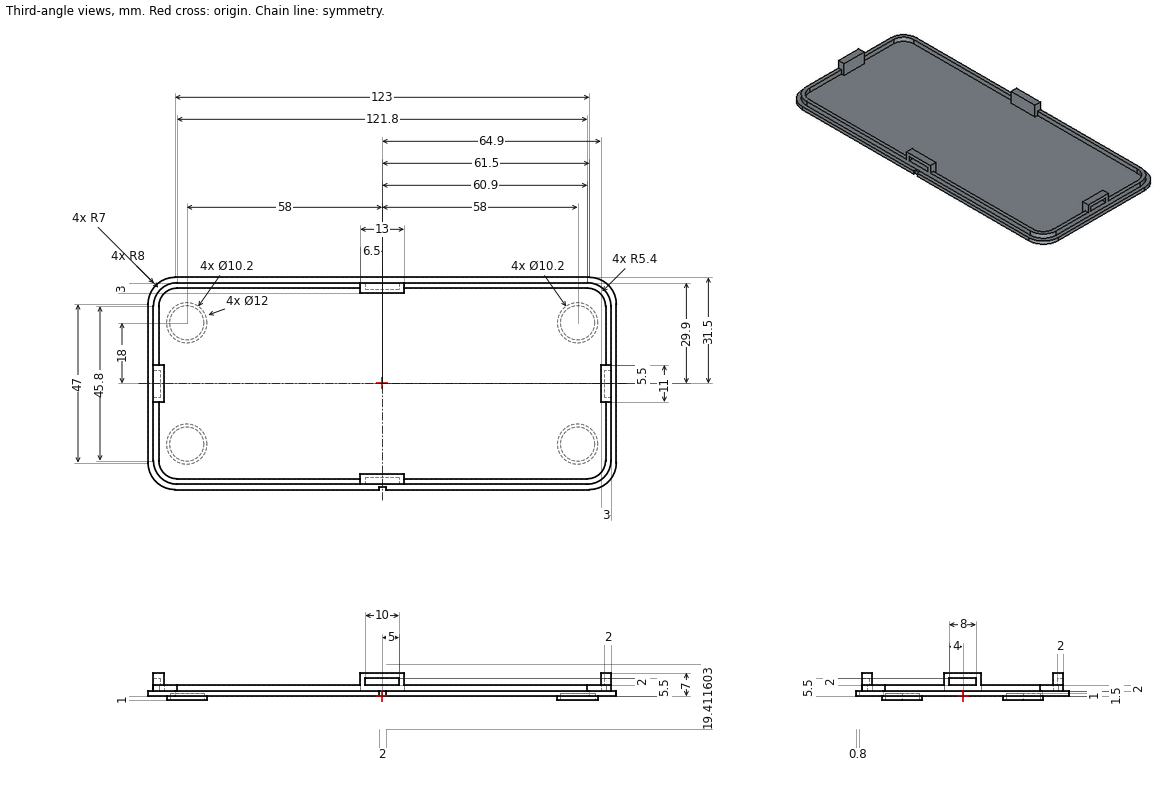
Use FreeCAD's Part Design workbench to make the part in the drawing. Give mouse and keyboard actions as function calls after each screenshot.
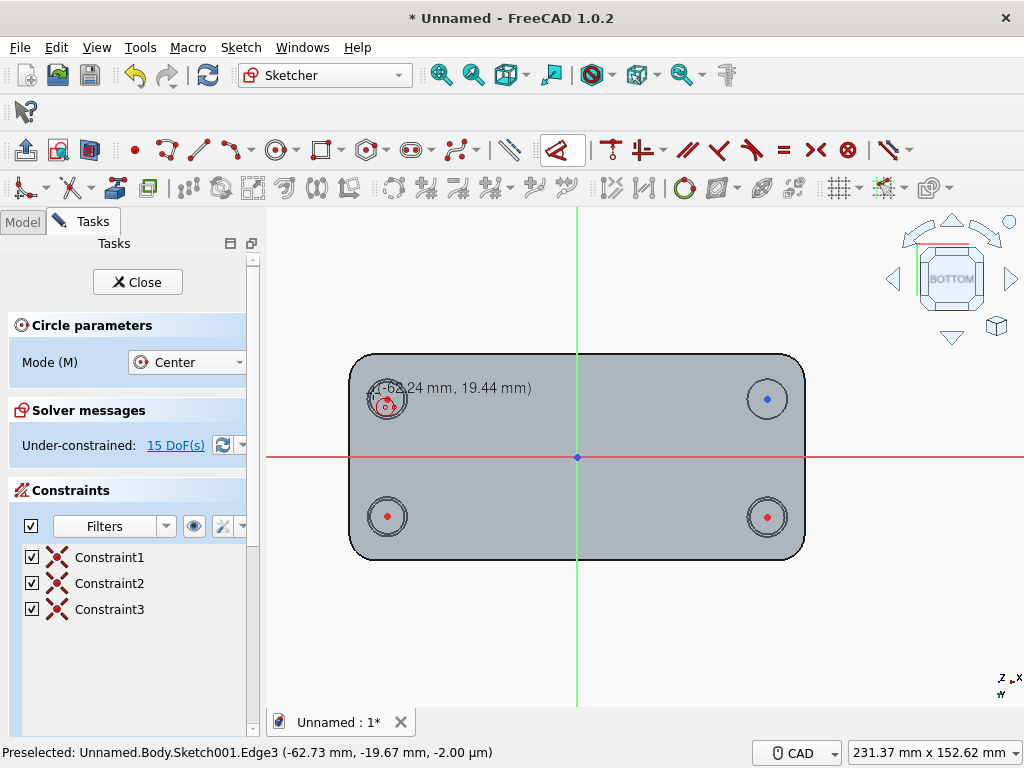
scroll(767, 398, up, 2)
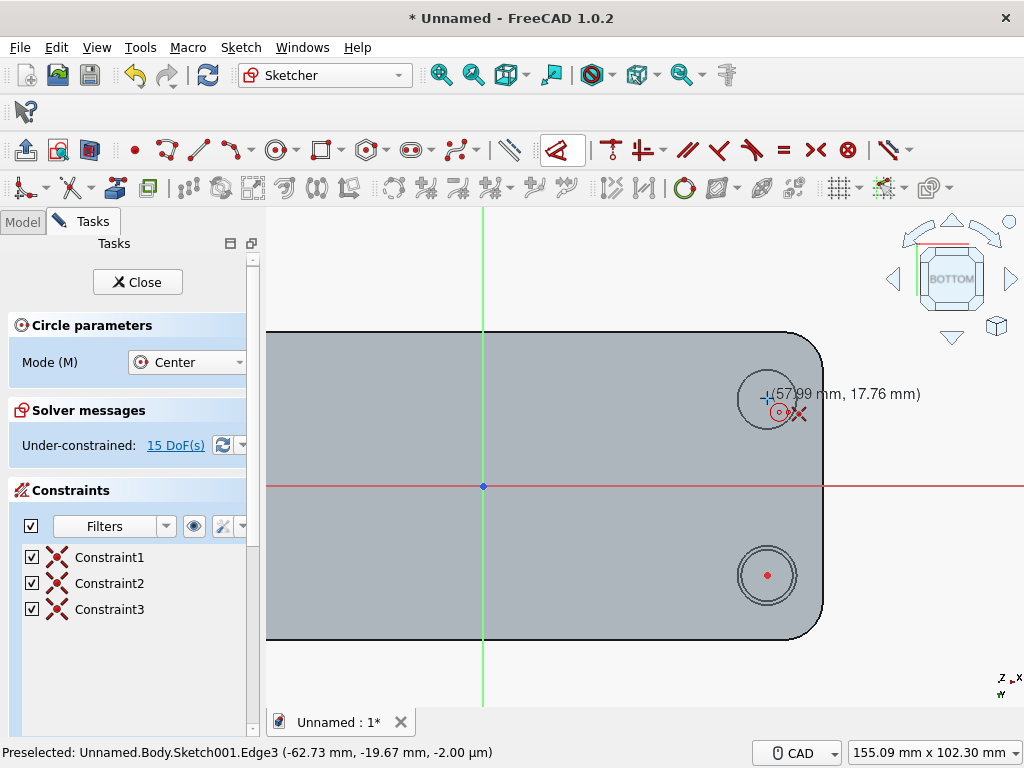
click(767, 399)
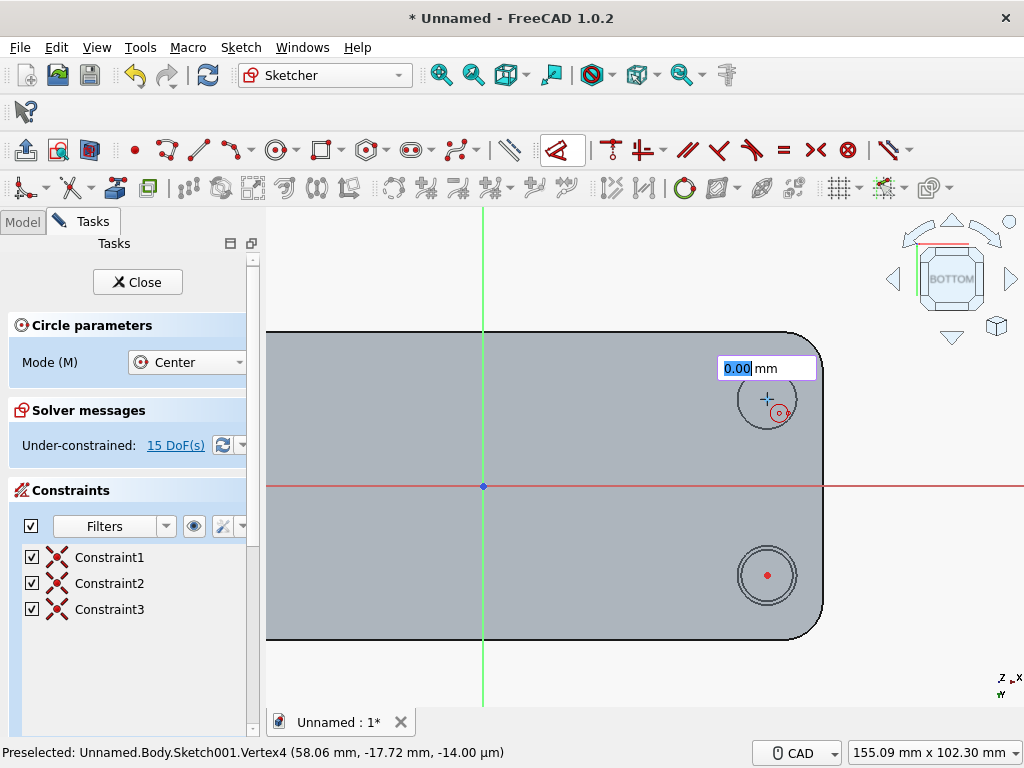
scroll(743, 390, up, 7)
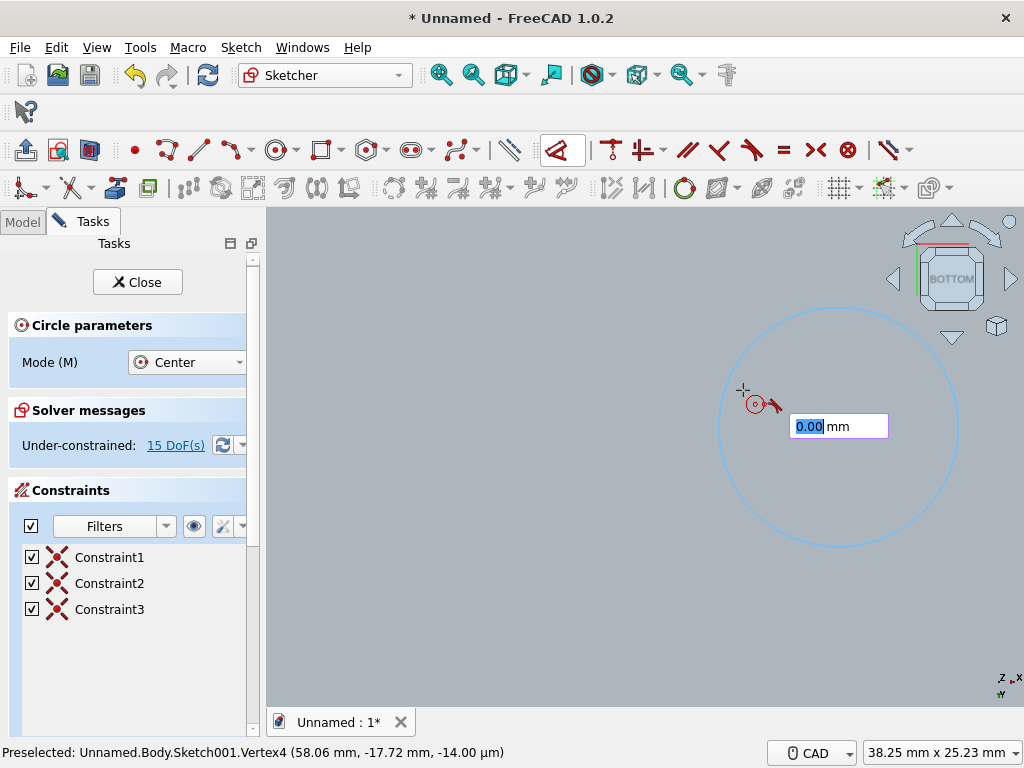
click(742, 387)
key(Escape)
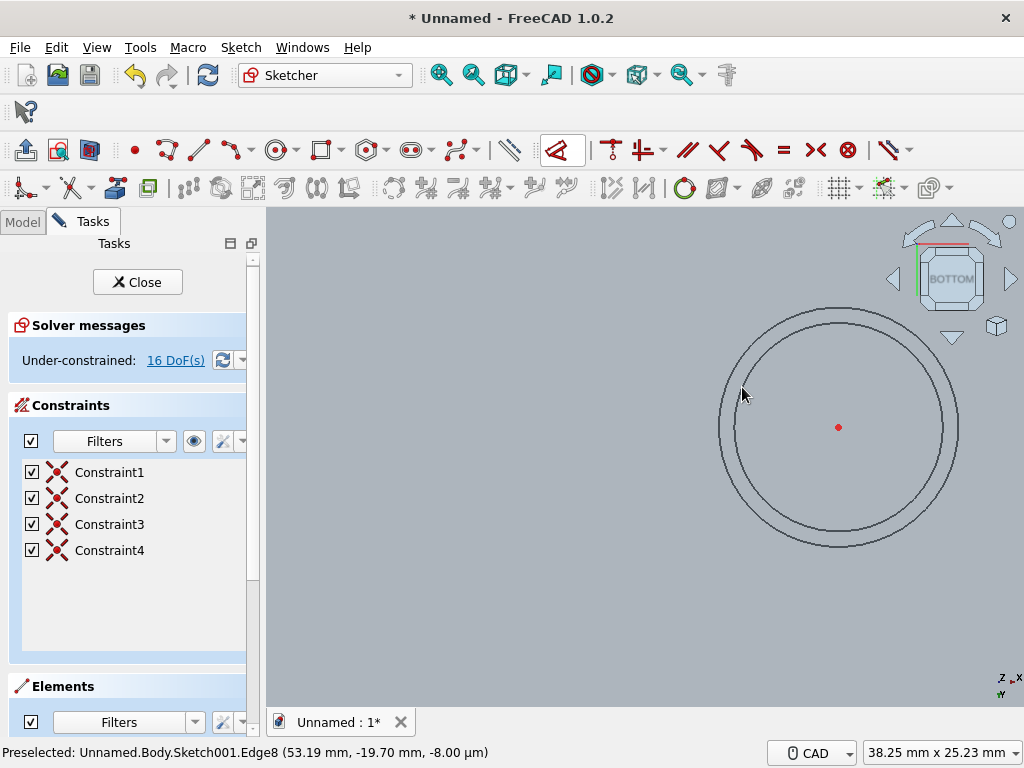
scroll(752, 393, down, 9)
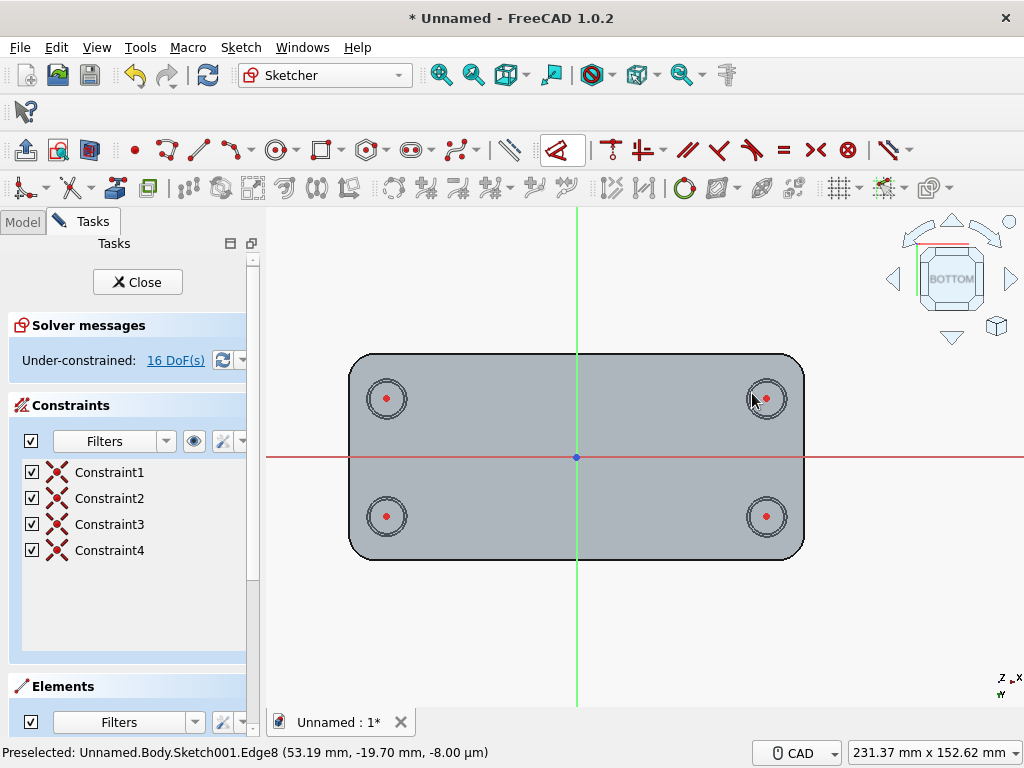
scroll(401, 503, up, 9)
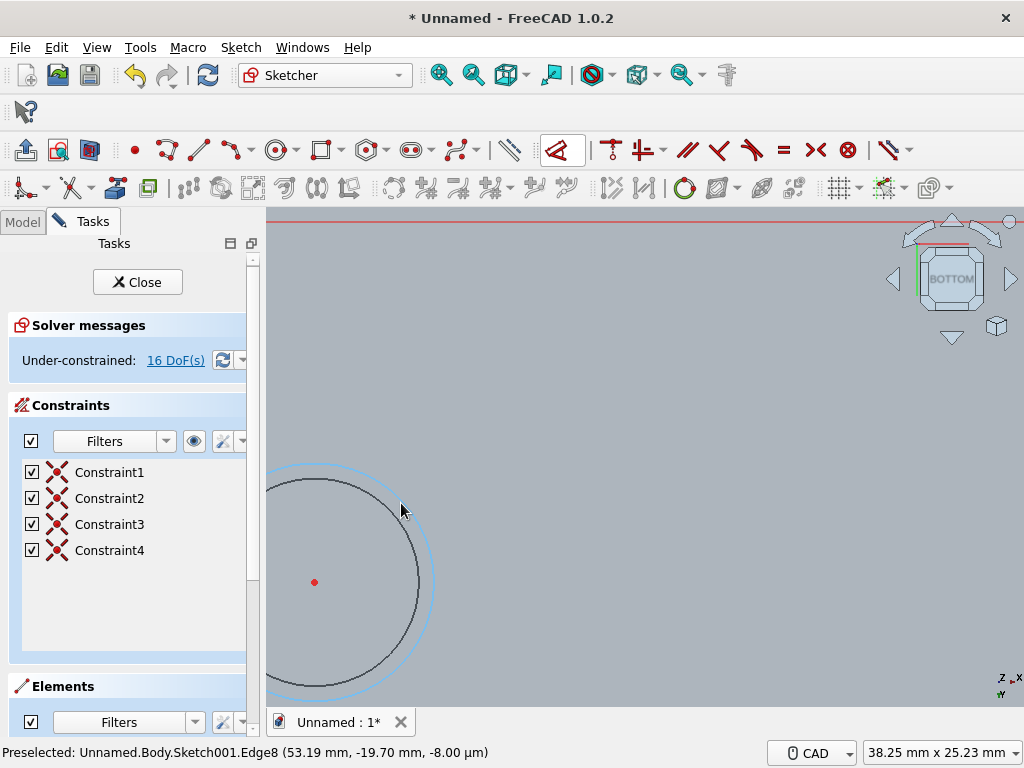
click(399, 498)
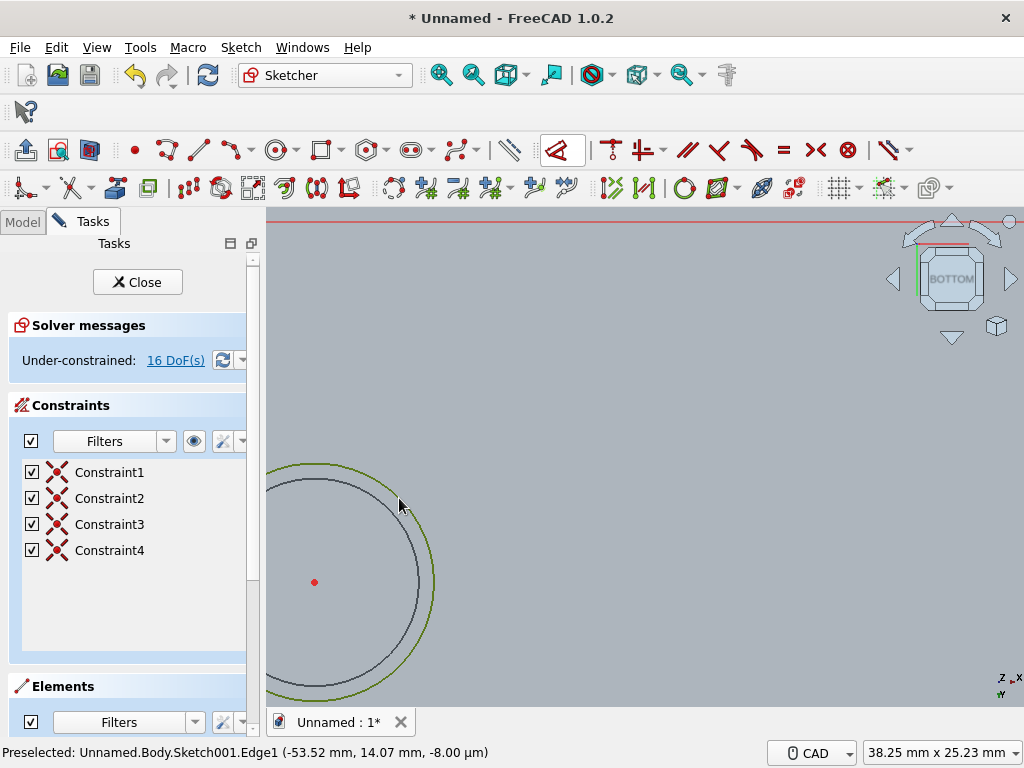
scroll(401, 504, down, 9)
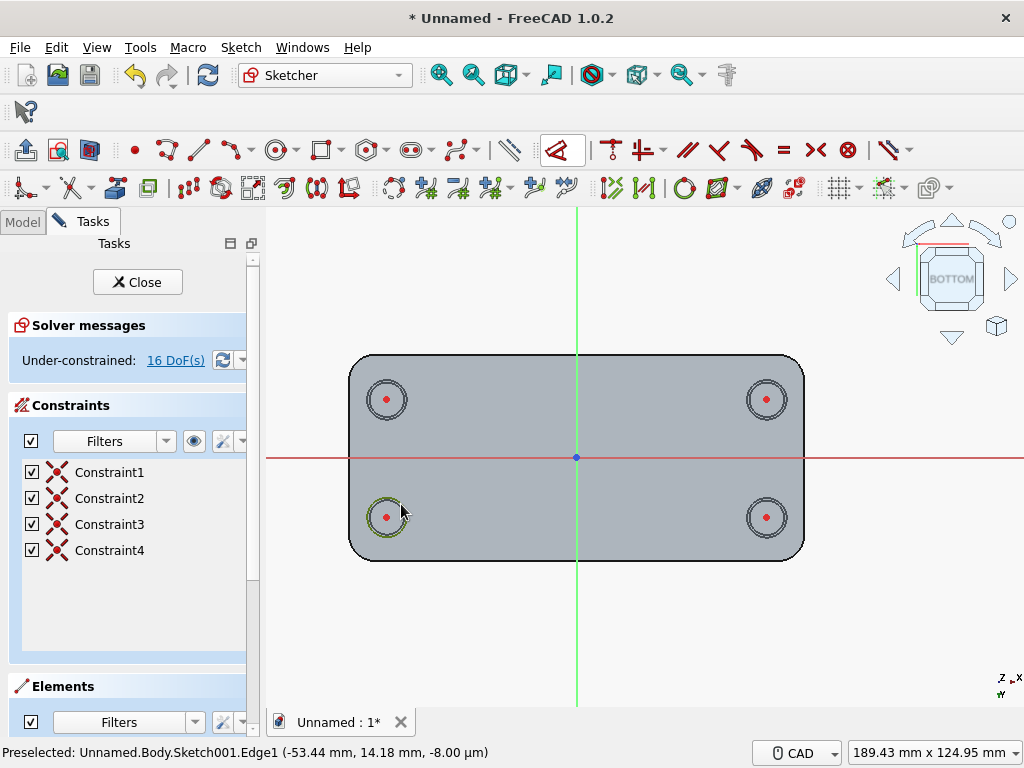
scroll(781, 504, up, 9)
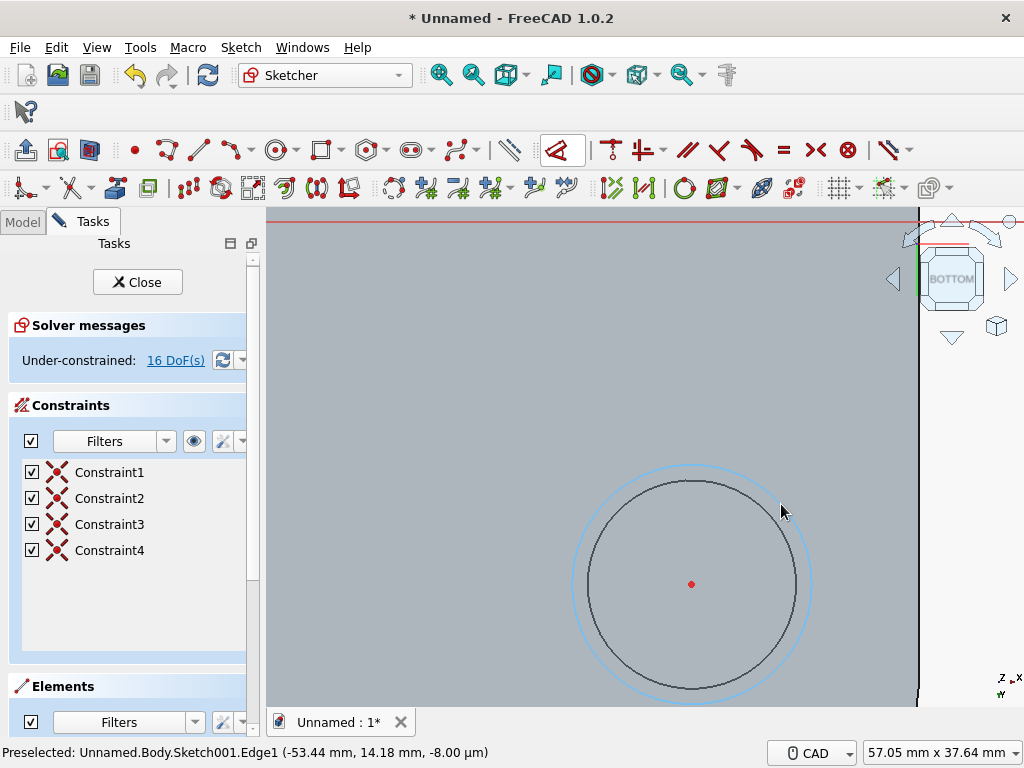
click(776, 500)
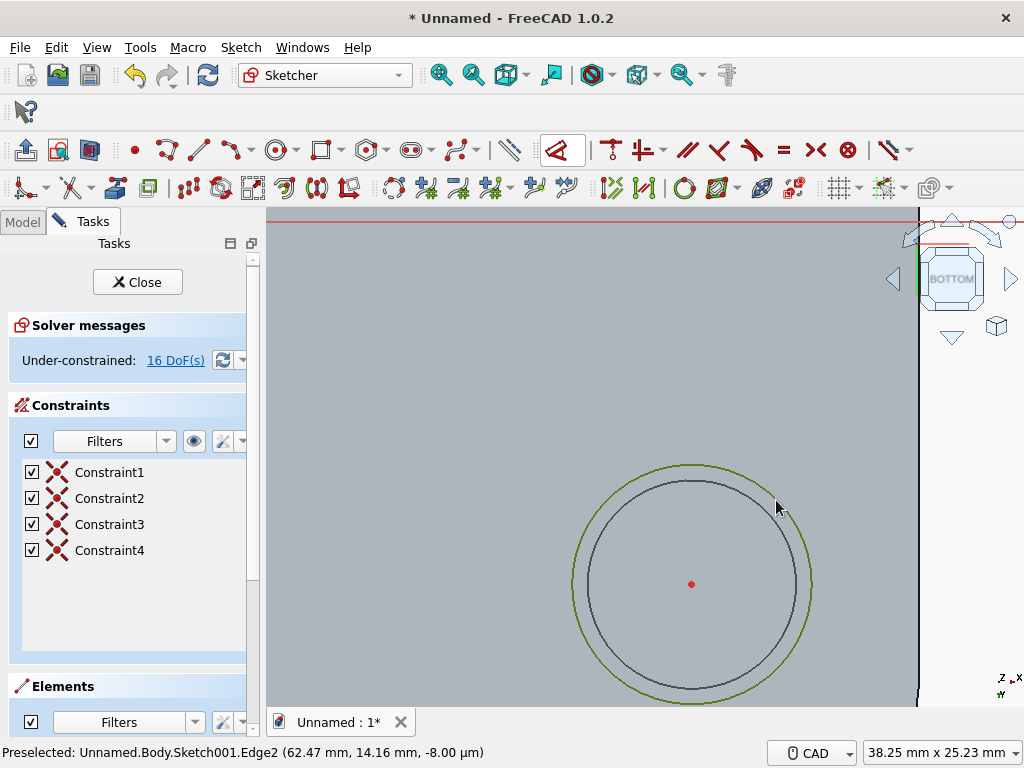
scroll(782, 504, down, 9)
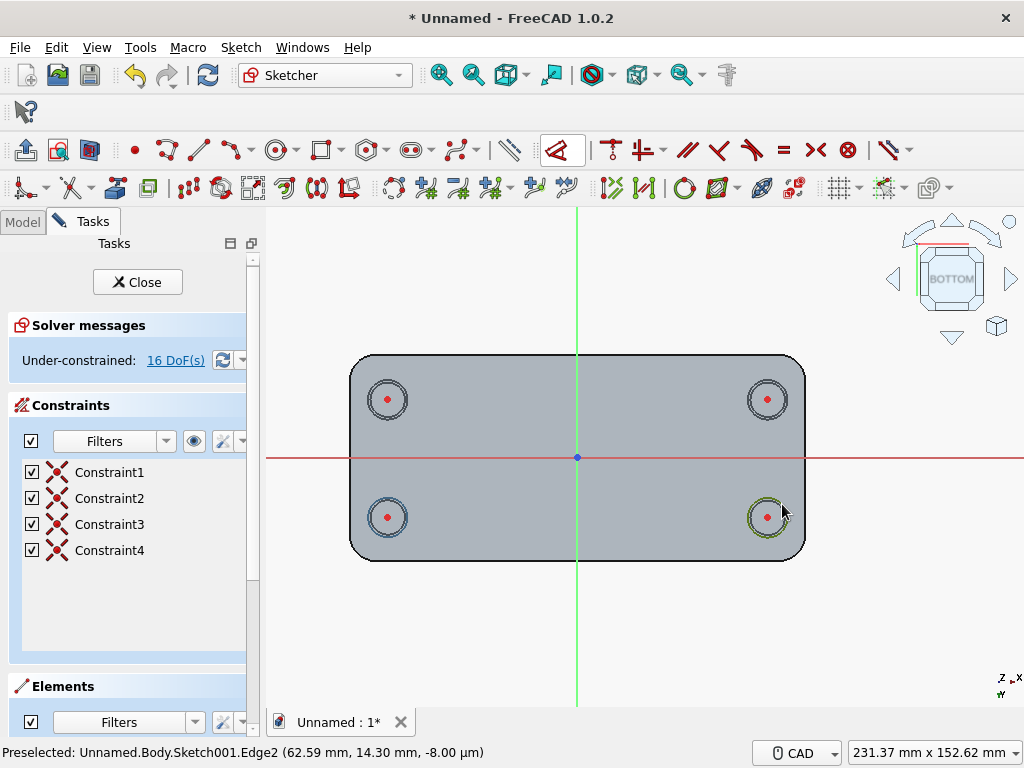
scroll(402, 386, up, 9)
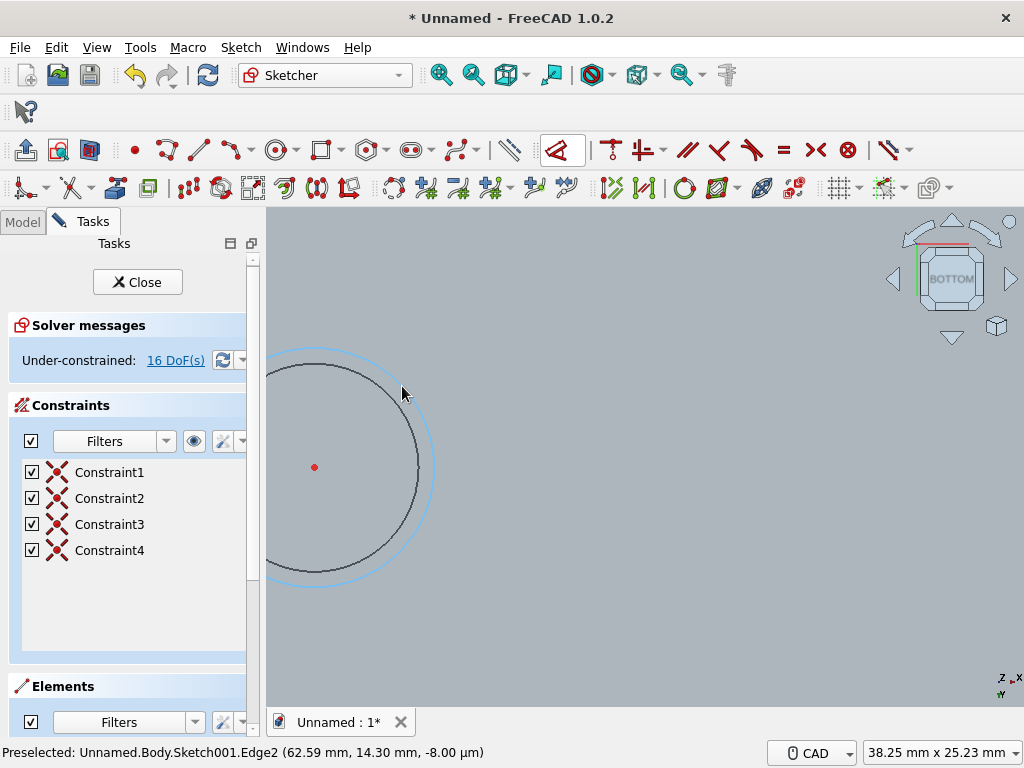
click(399, 383)